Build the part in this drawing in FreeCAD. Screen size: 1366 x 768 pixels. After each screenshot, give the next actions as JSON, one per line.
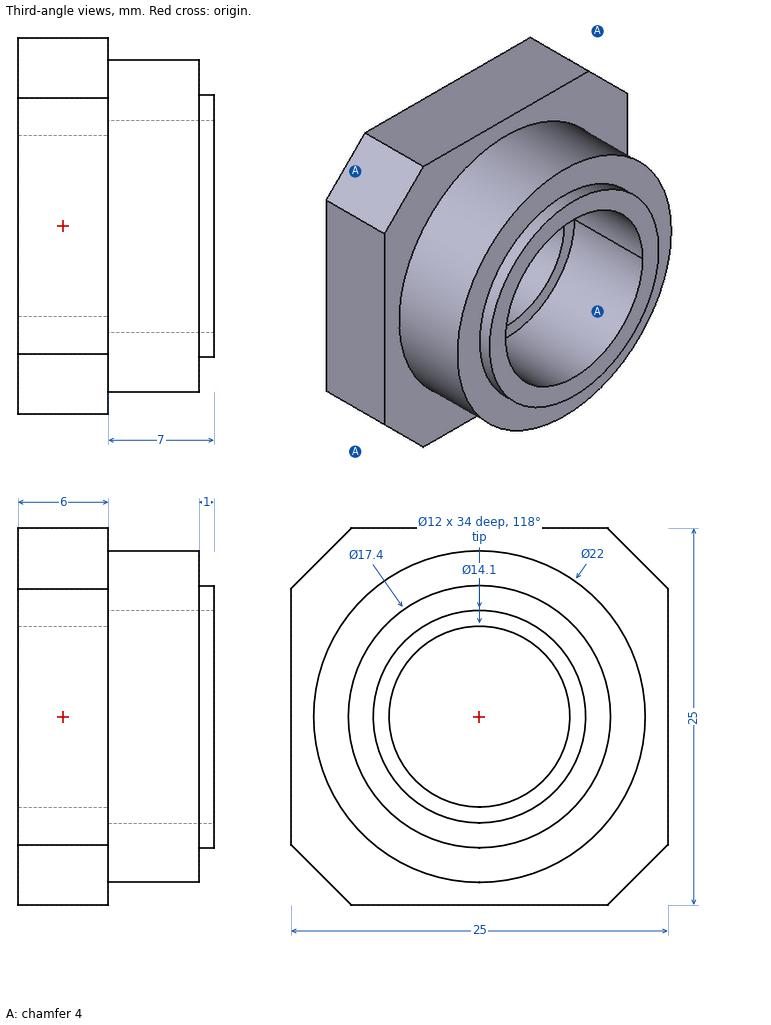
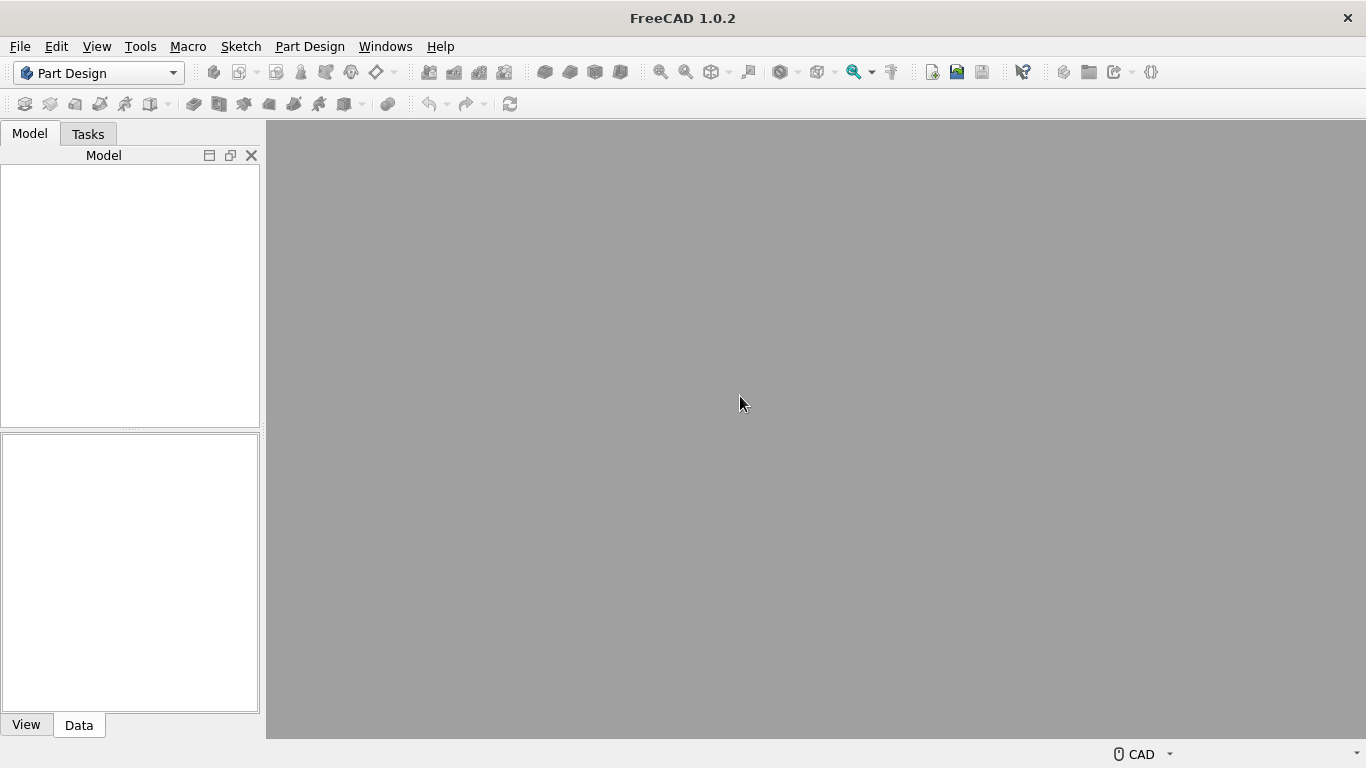
{"action": "left_click", "coordinate": [932, 72]}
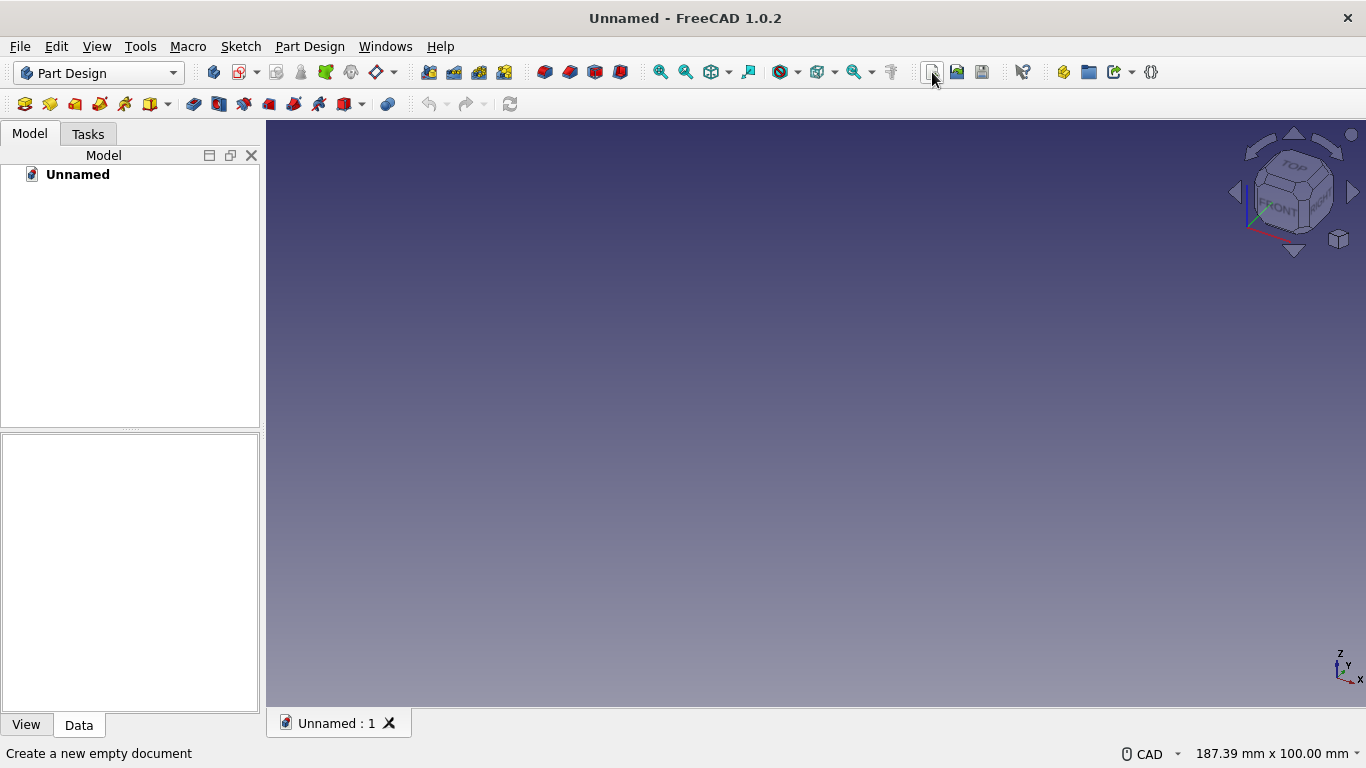
{"action": "left_click", "coordinate": [238, 72]}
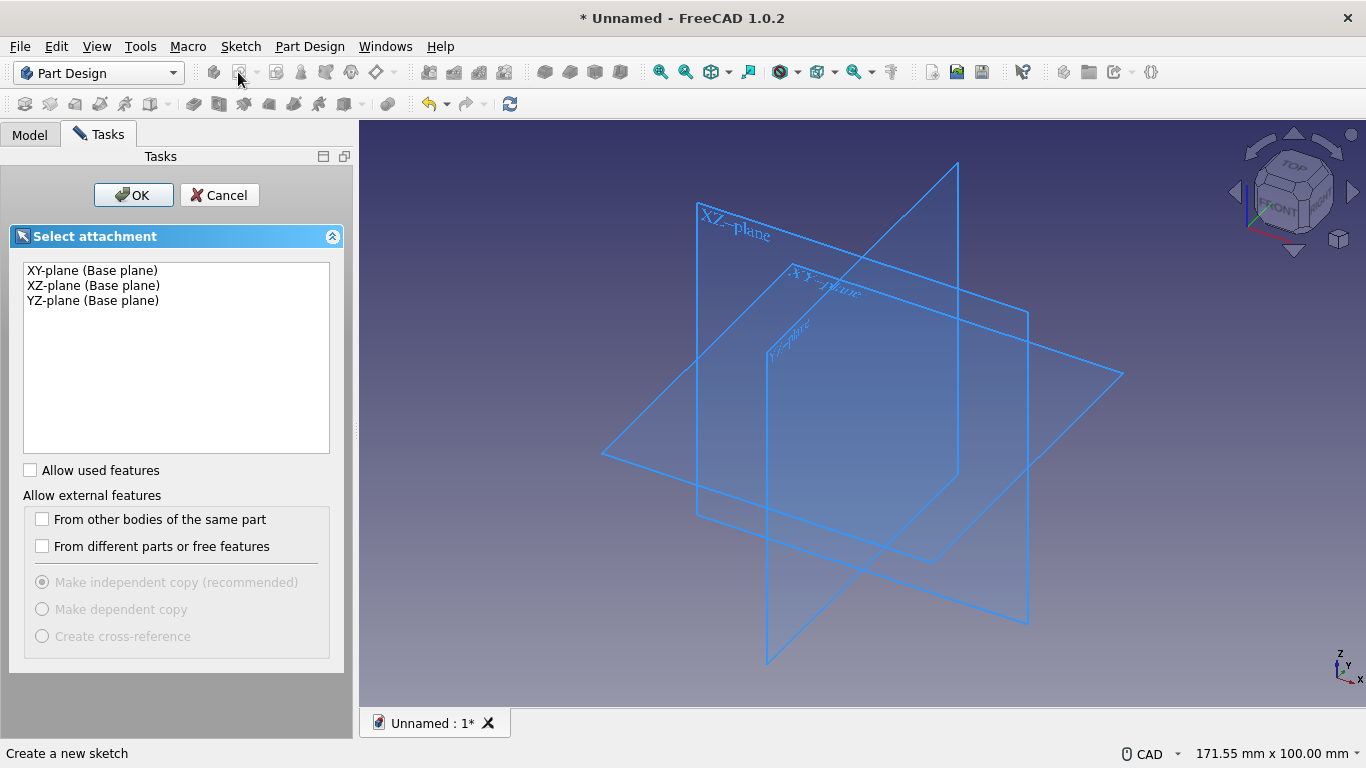
{"action": "left_click", "coordinate": [84, 300]}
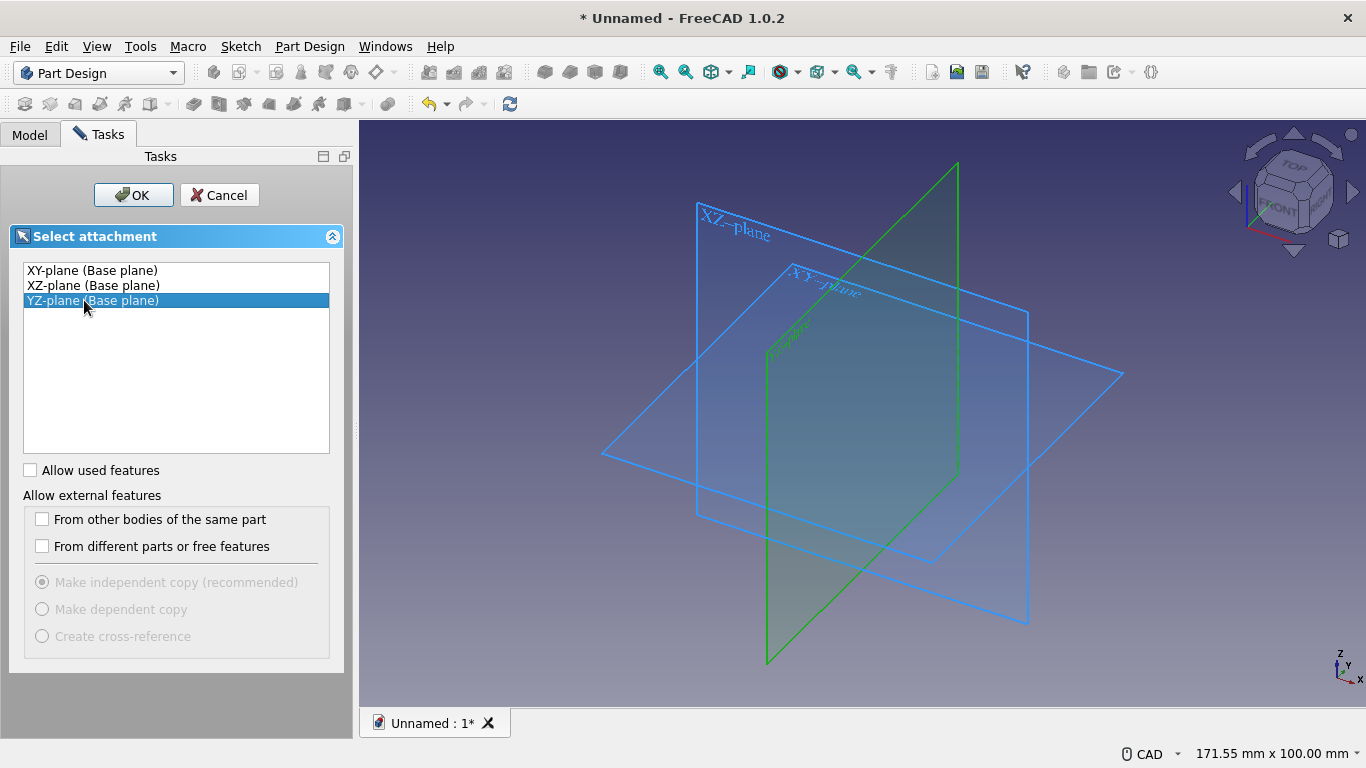
{"action": "left_click", "coordinate": [134, 195]}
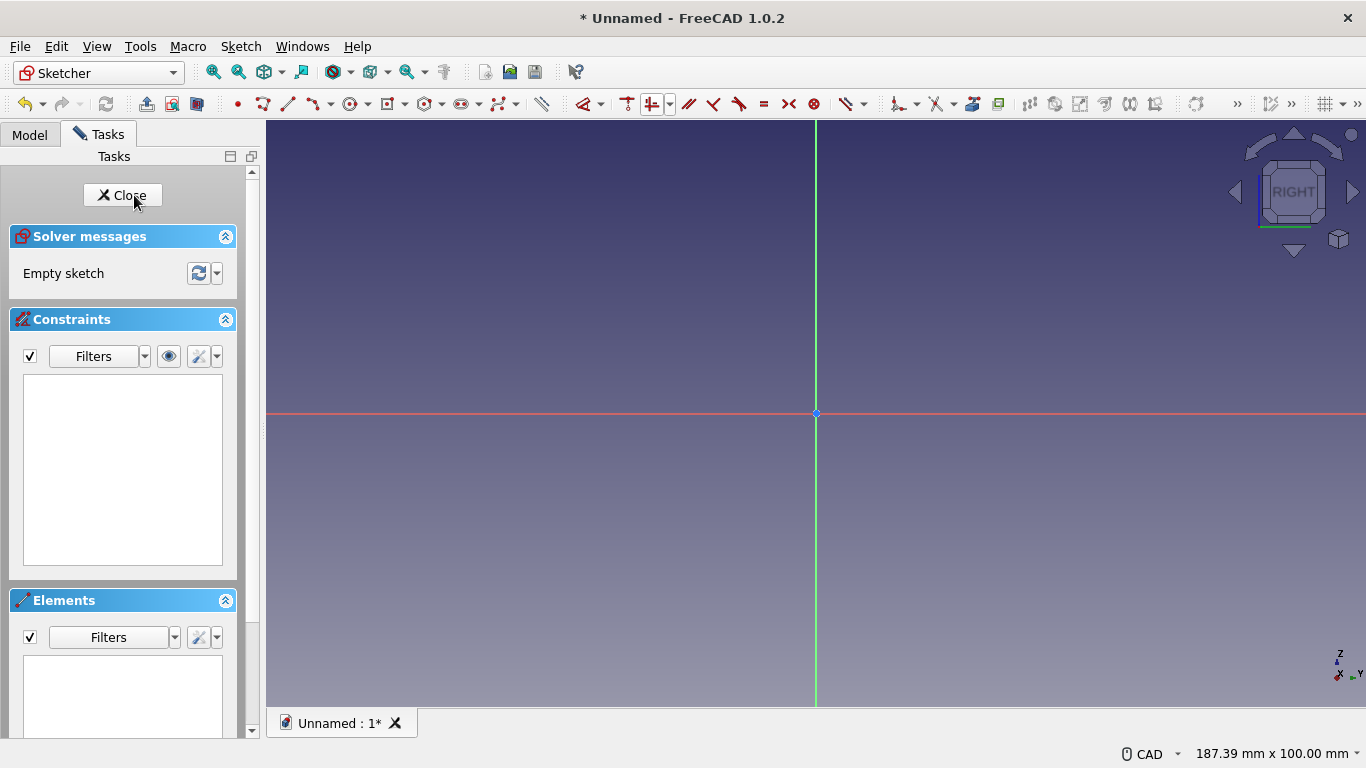
{"action": "scroll", "coordinate": [856, 414], "scroll_direction": "up", "scroll_amount": 5}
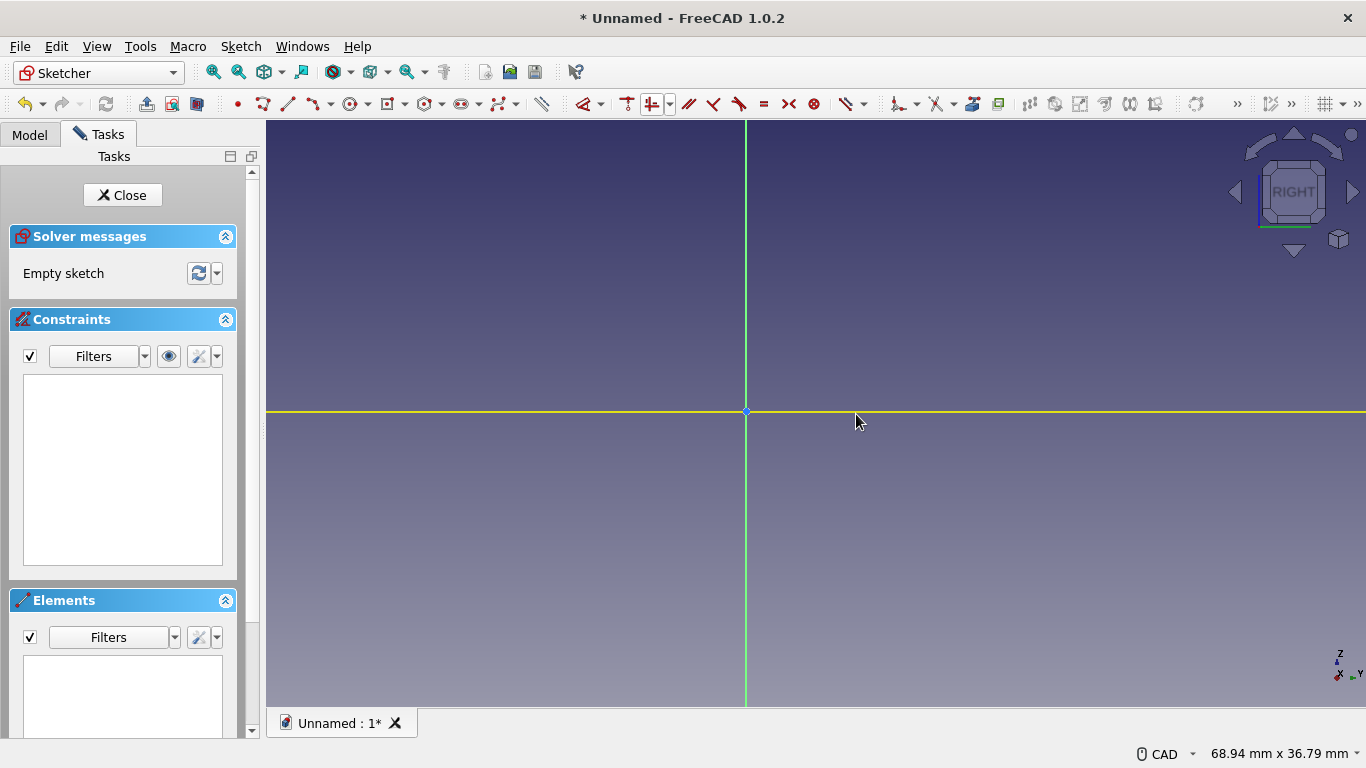
{"action": "left_click", "coordinate": [386, 104]}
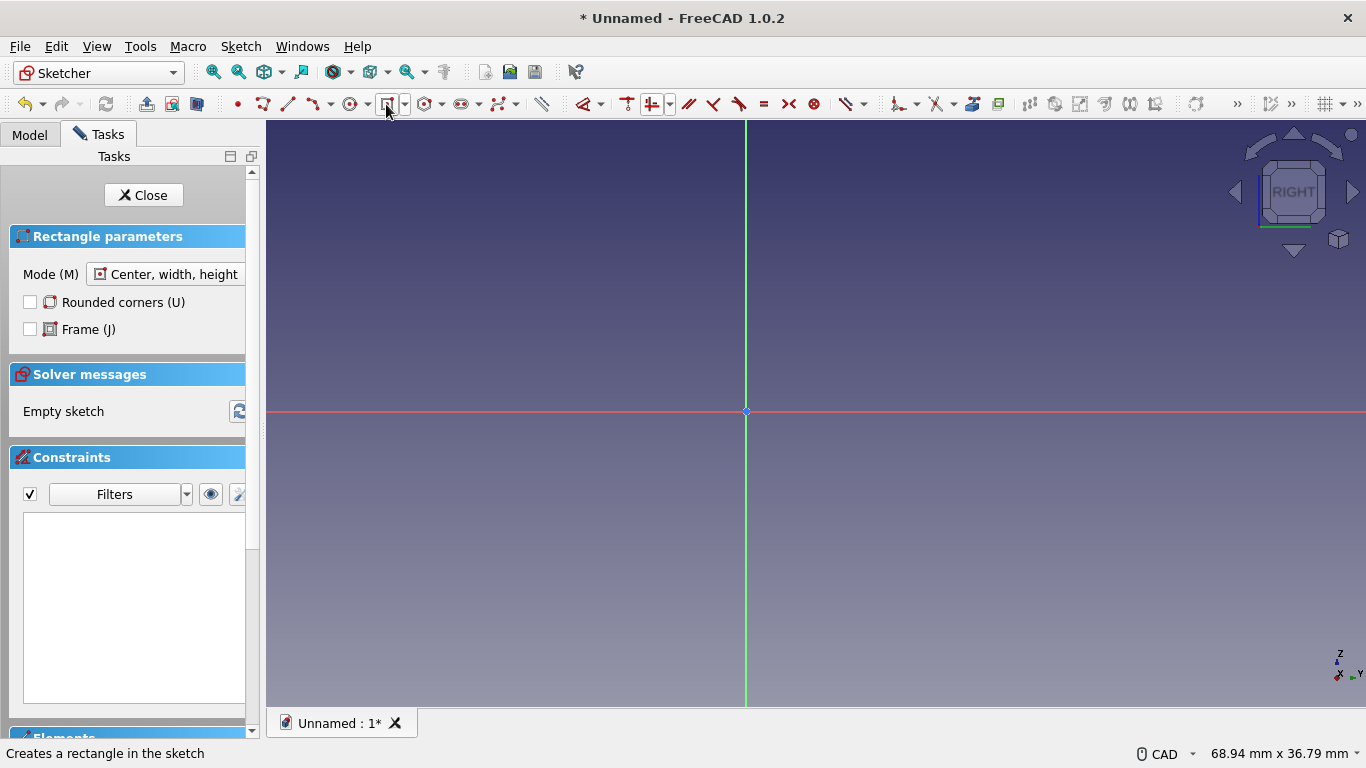
{"action": "left_click", "coordinate": [746, 412]}
{"action": "mouse_move", "coordinate": [946, 212]}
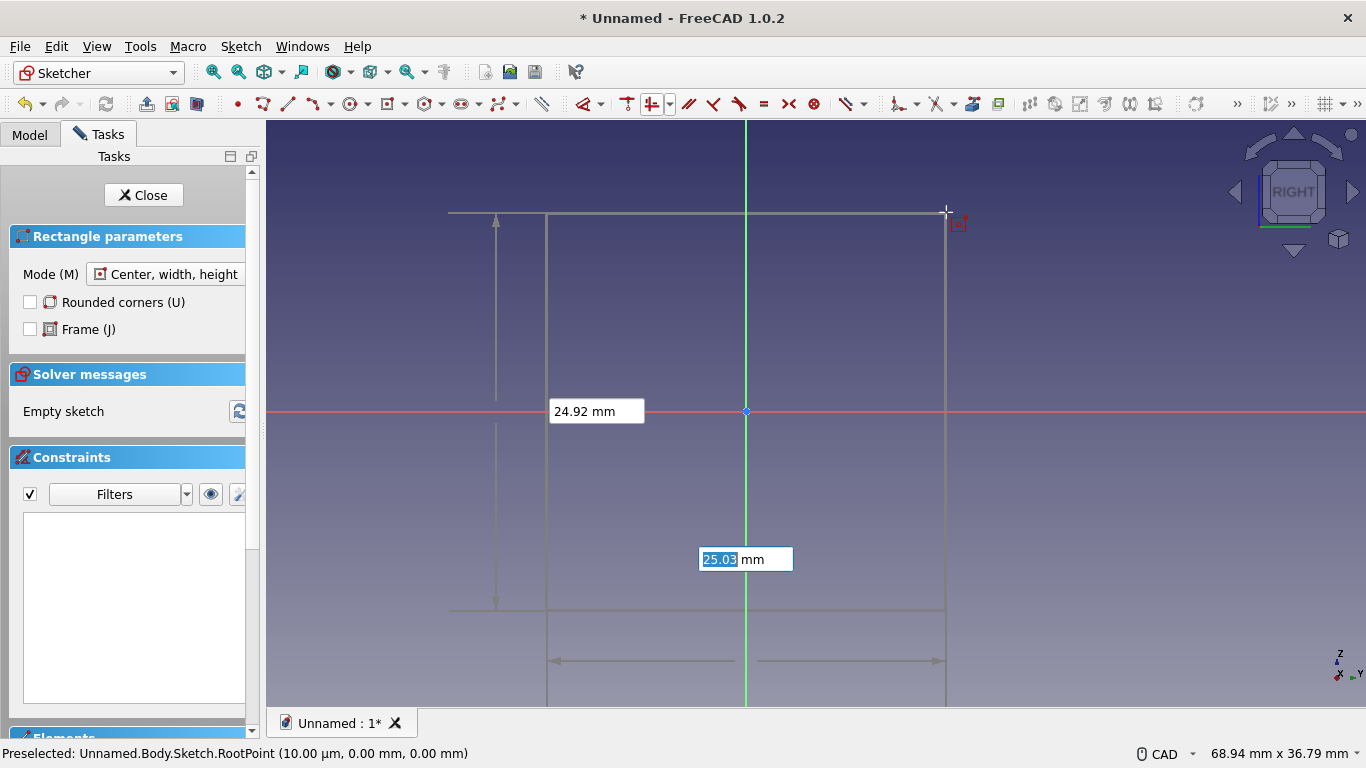
{"action": "type", "text": "25"}
{"action": "key", "text": "Tab"}
{"action": "type", "text": "25"}
{"action": "key", "text": "Return"}
{"action": "key", "text": "Escape"}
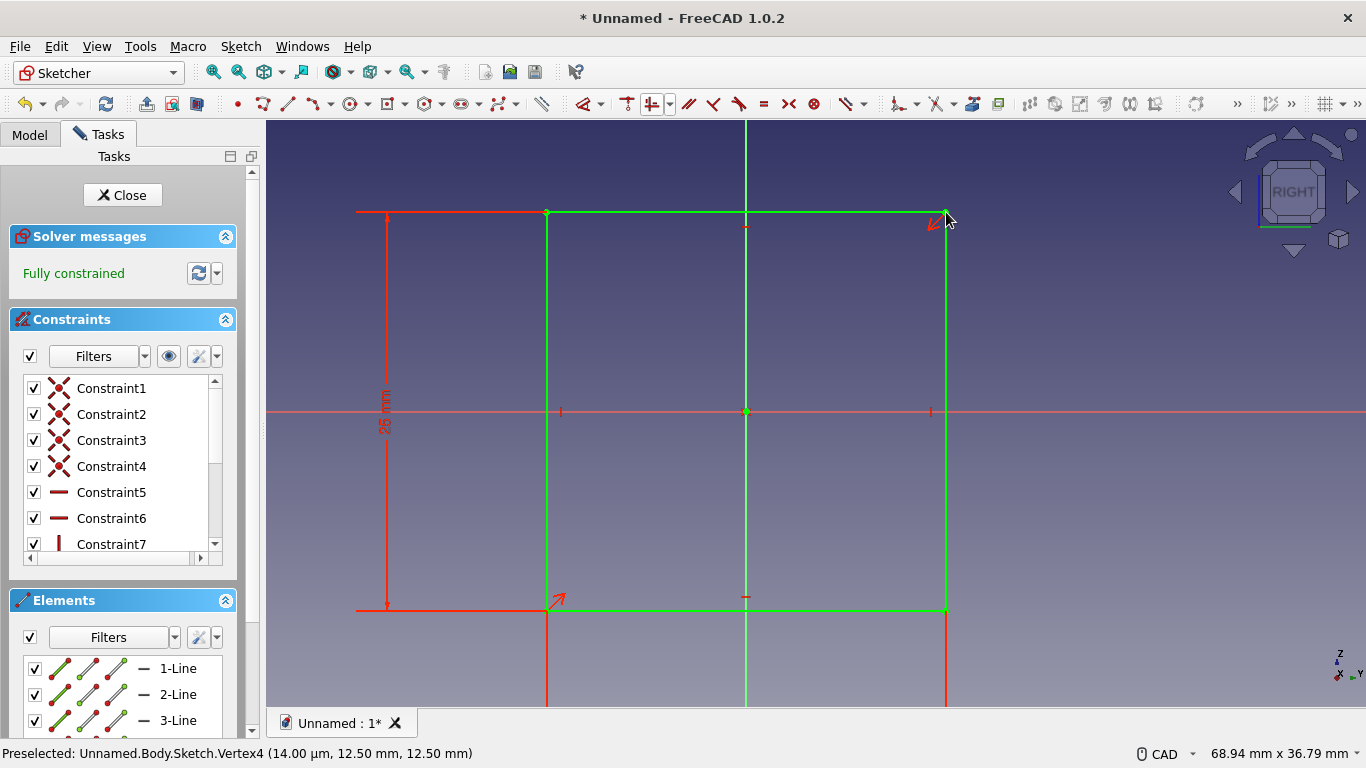
{"action": "left_click", "coordinate": [123, 195]}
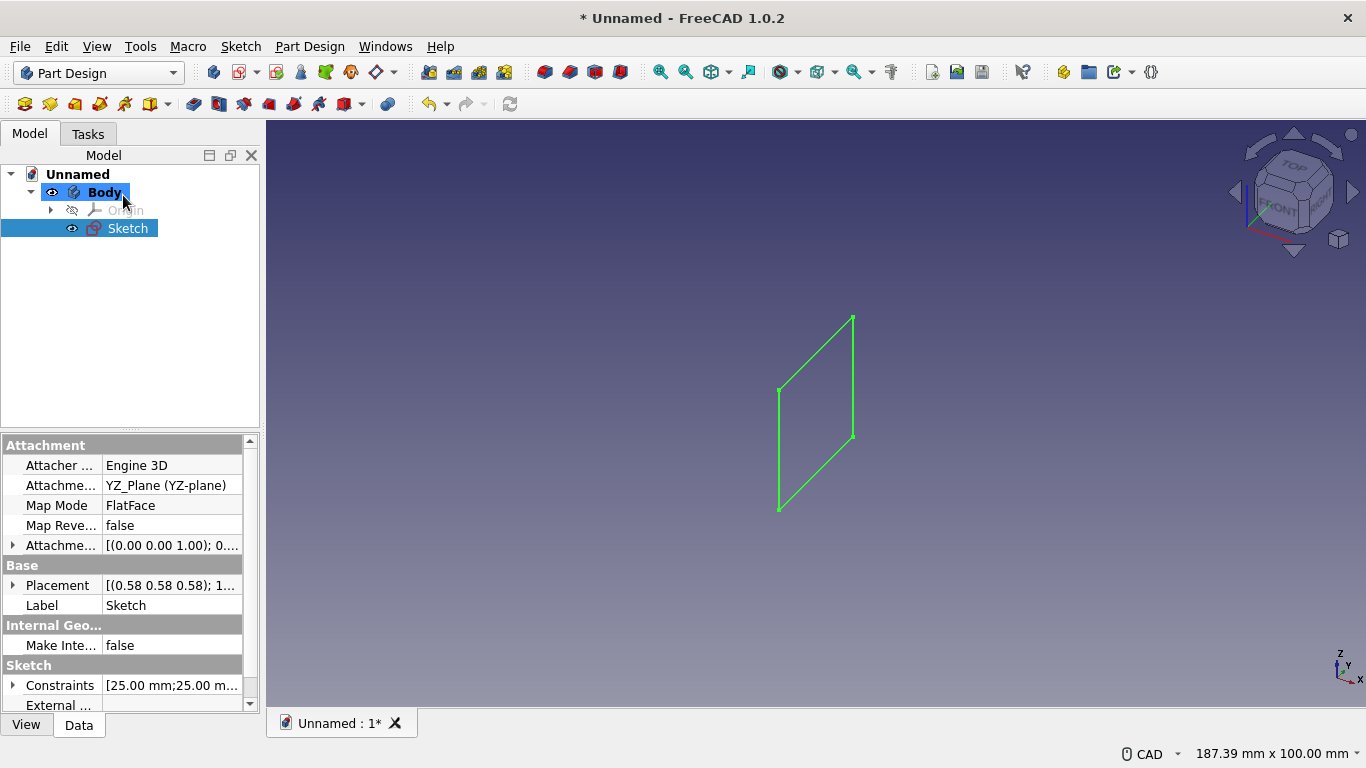
{"action": "left_click", "coordinate": [25, 104]}